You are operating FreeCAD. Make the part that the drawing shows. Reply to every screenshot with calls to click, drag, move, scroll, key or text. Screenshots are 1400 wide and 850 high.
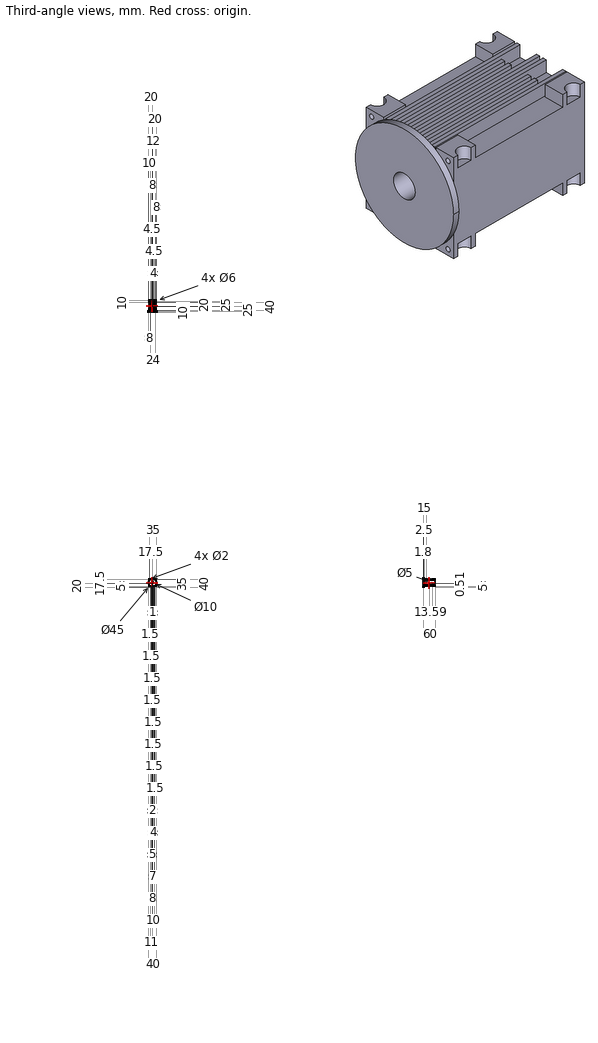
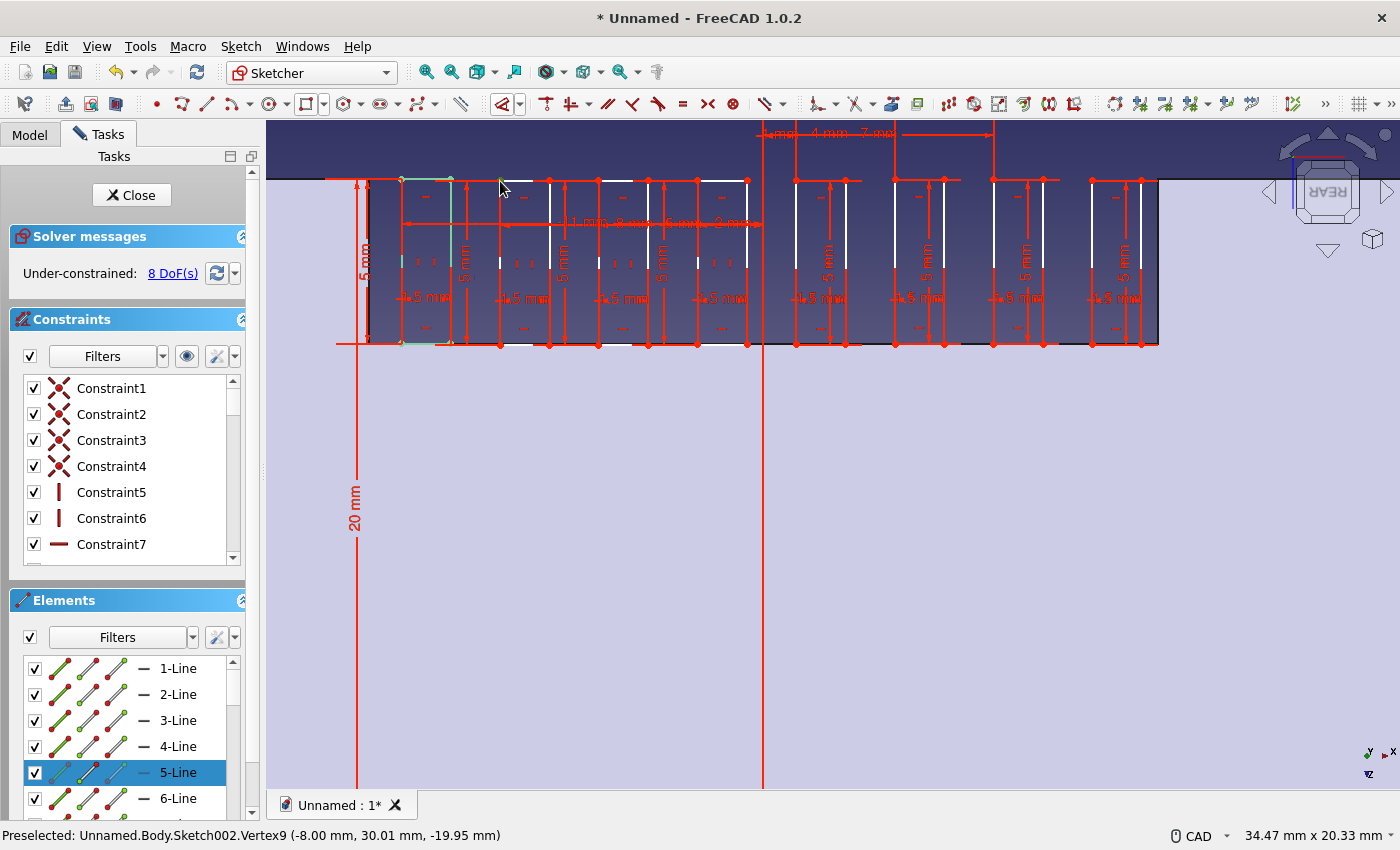
key(i)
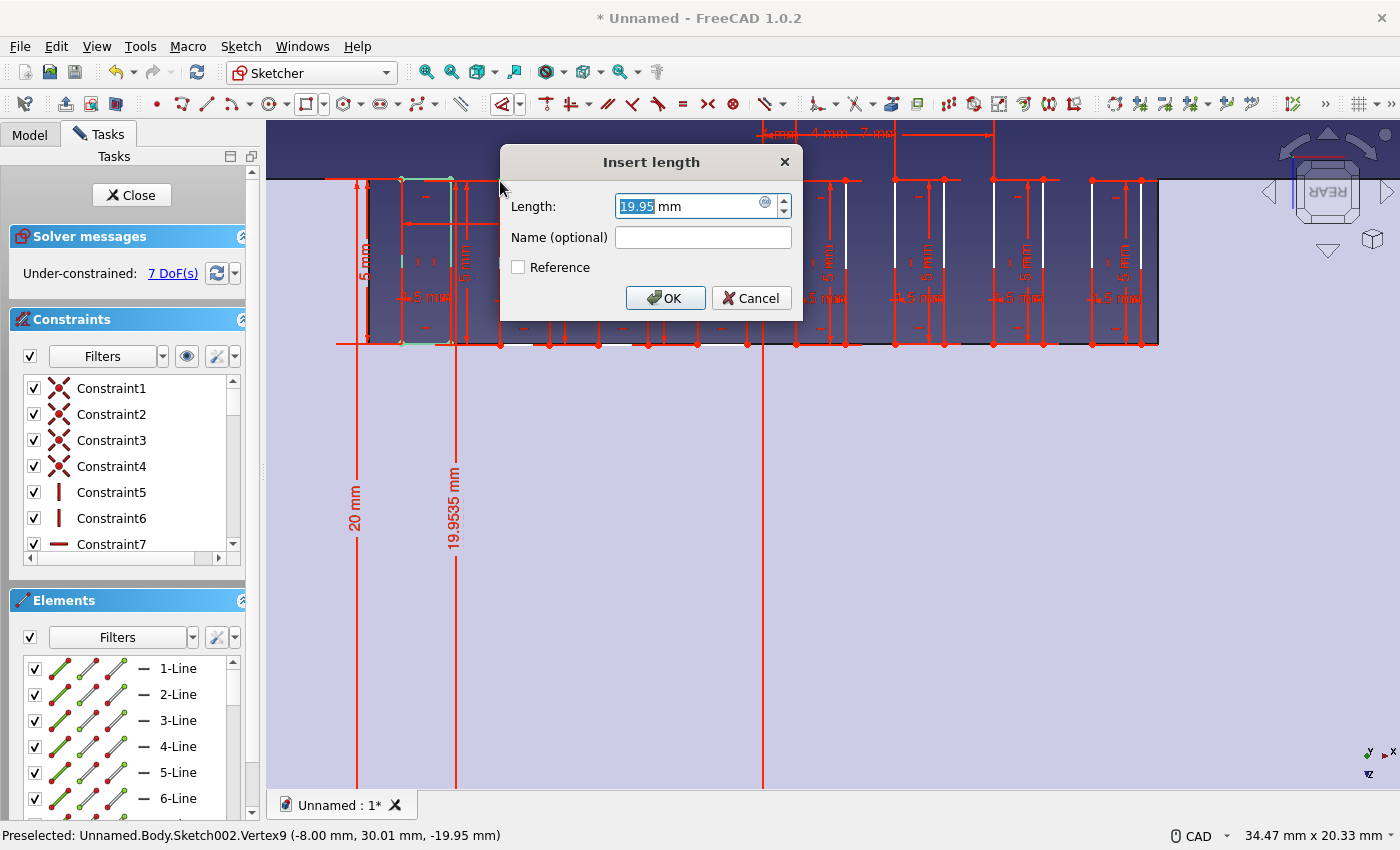
text(20)
key(Return)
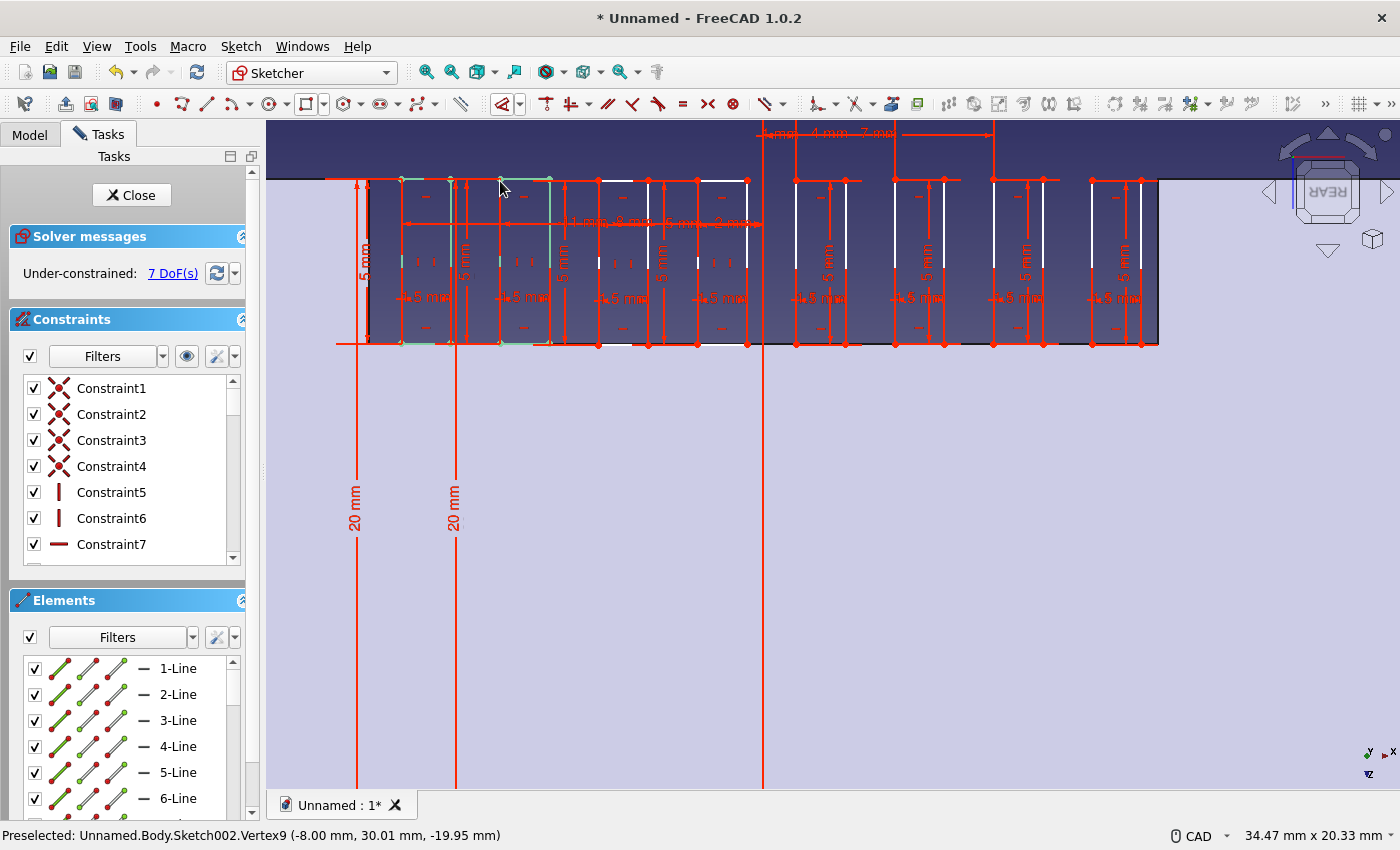
click(599, 181)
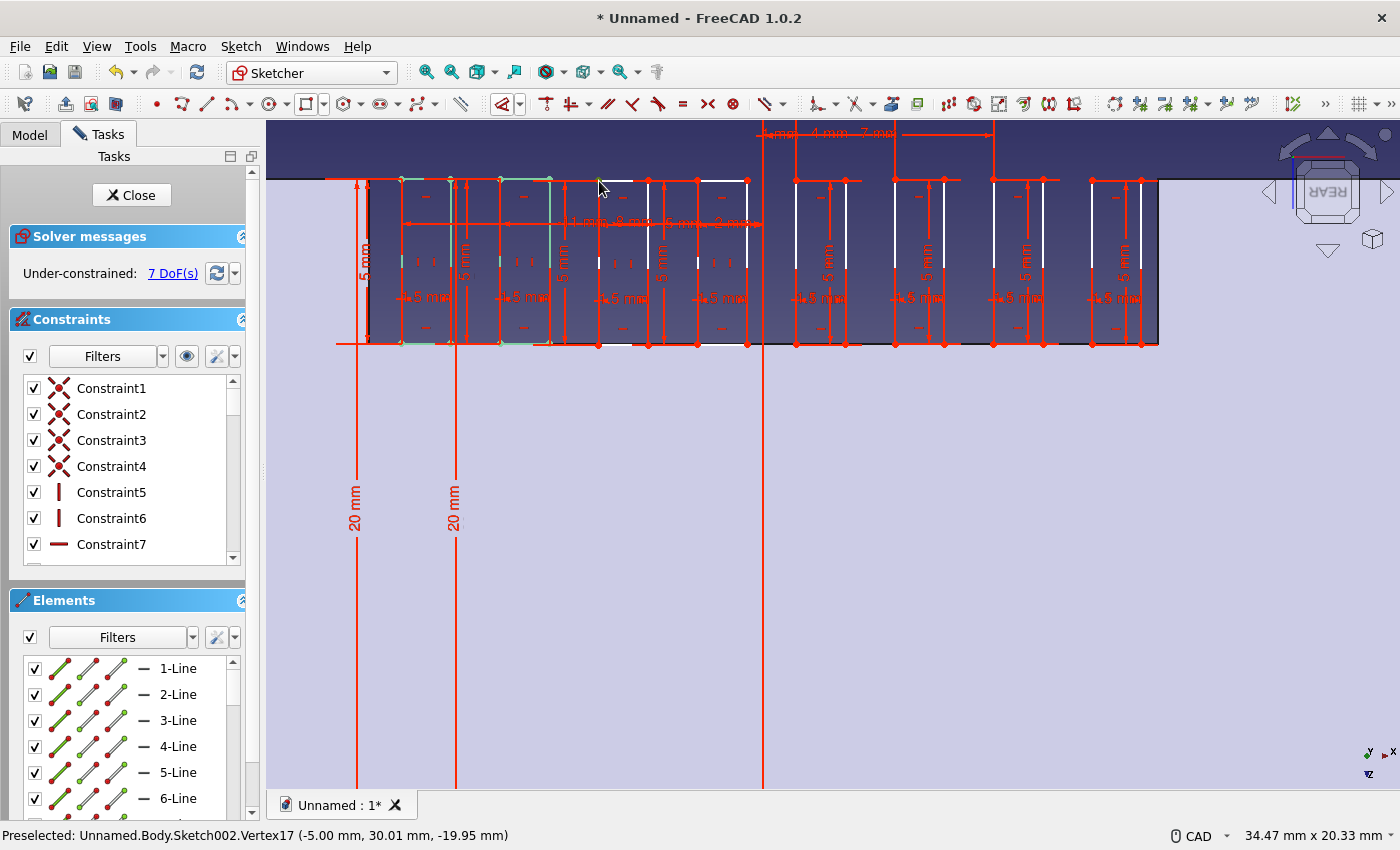
click(520, 104)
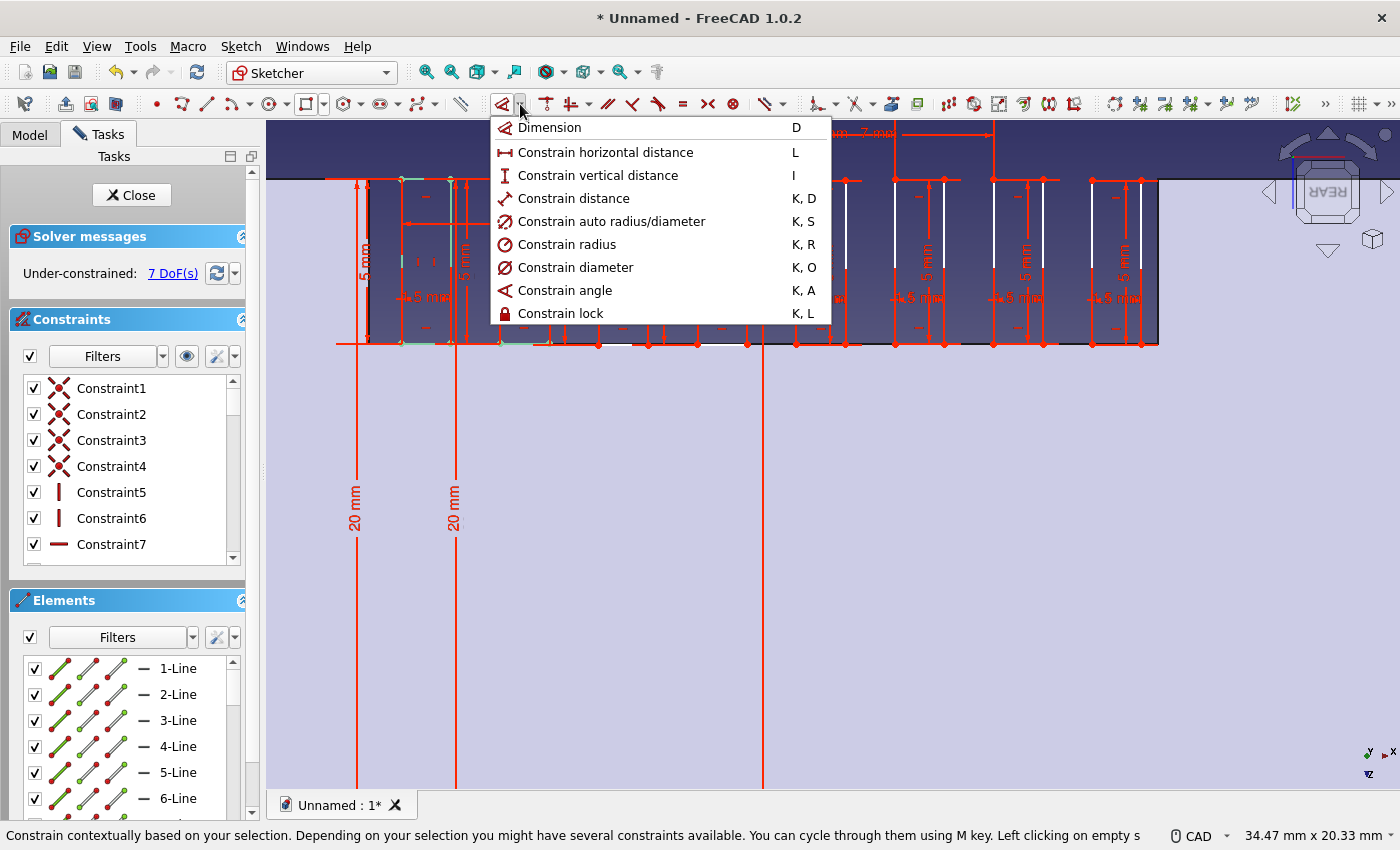
click(661, 176)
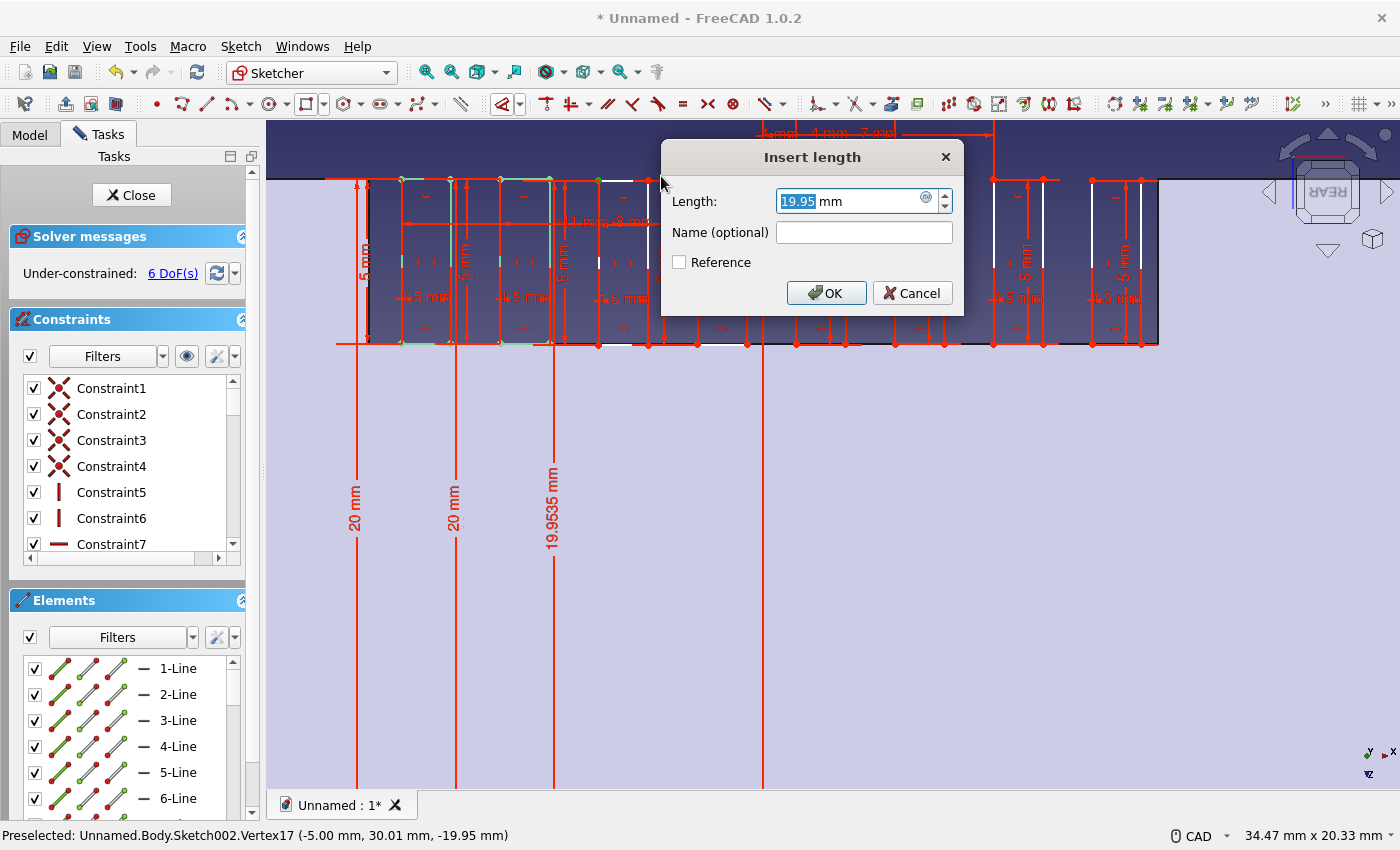
text(20)
key(Return)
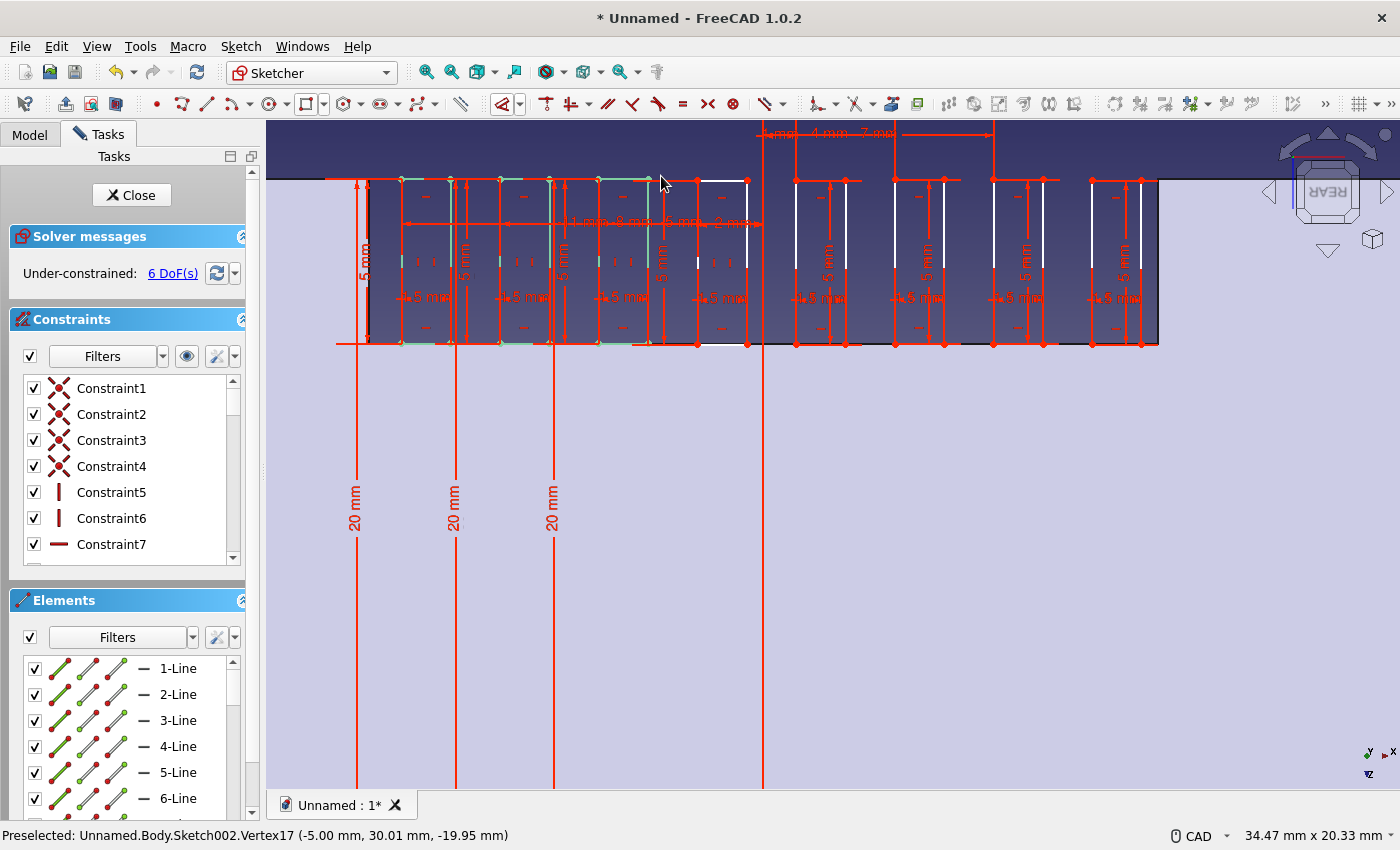
click(698, 181)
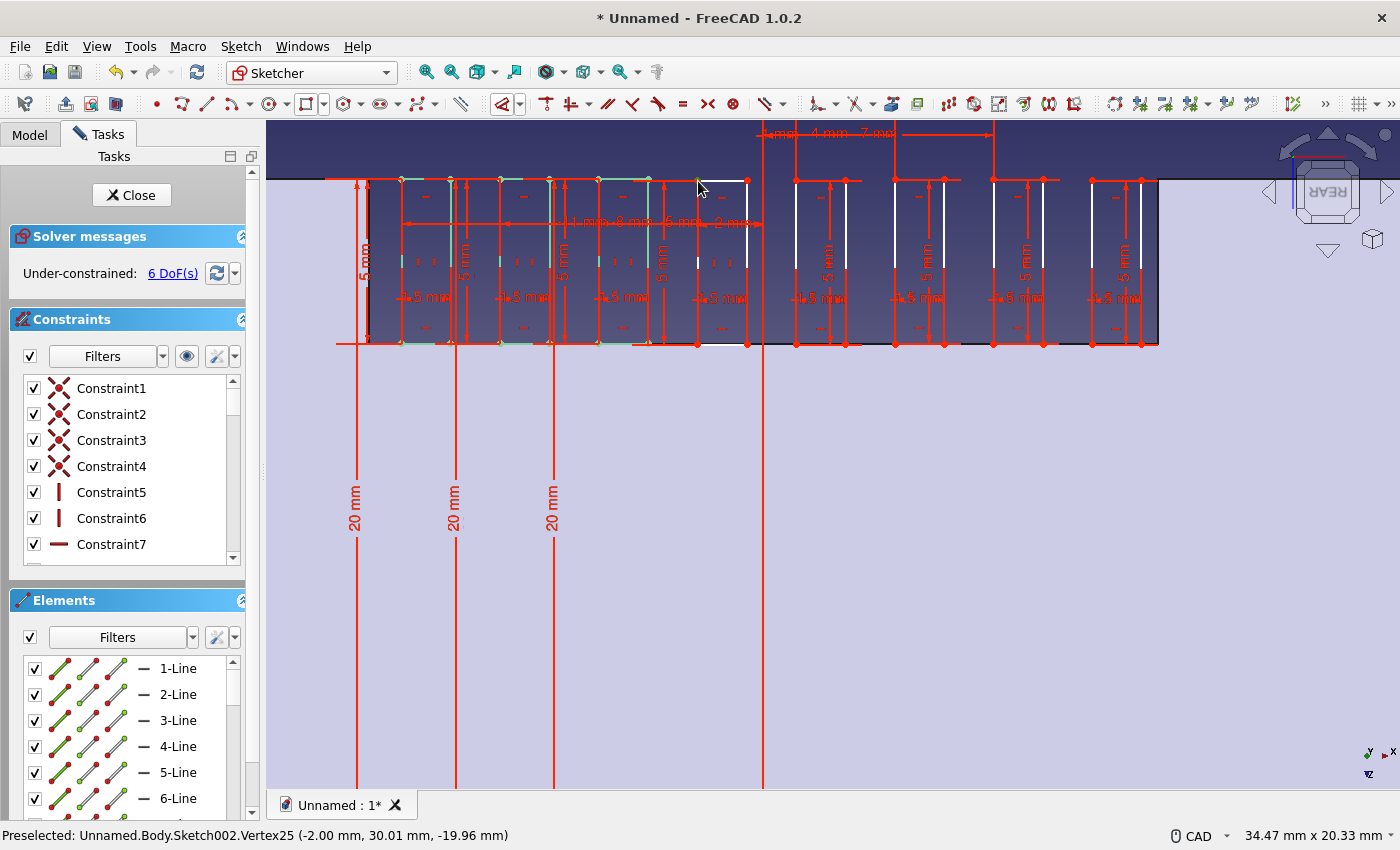
click(520, 104)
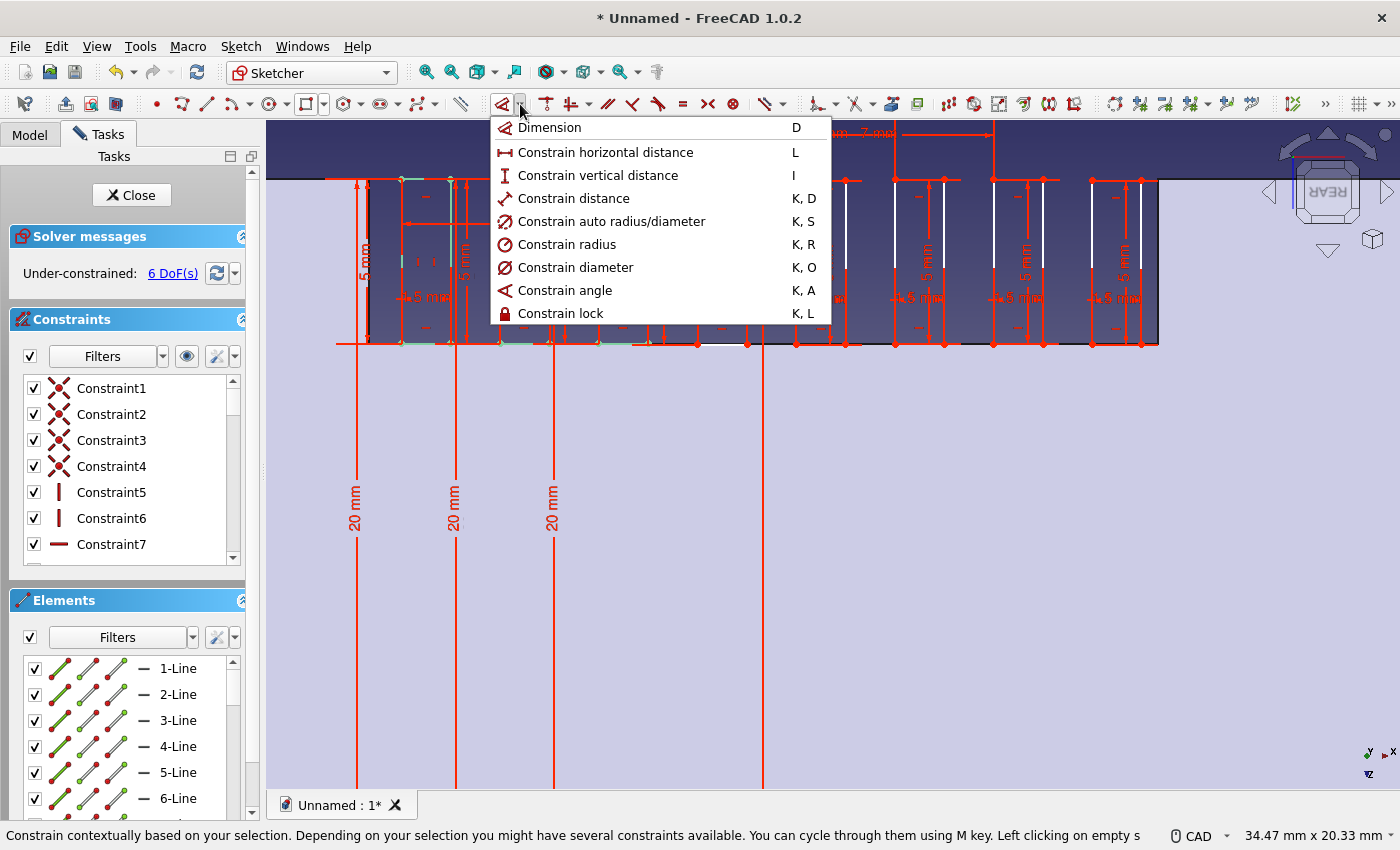
click(661, 176)